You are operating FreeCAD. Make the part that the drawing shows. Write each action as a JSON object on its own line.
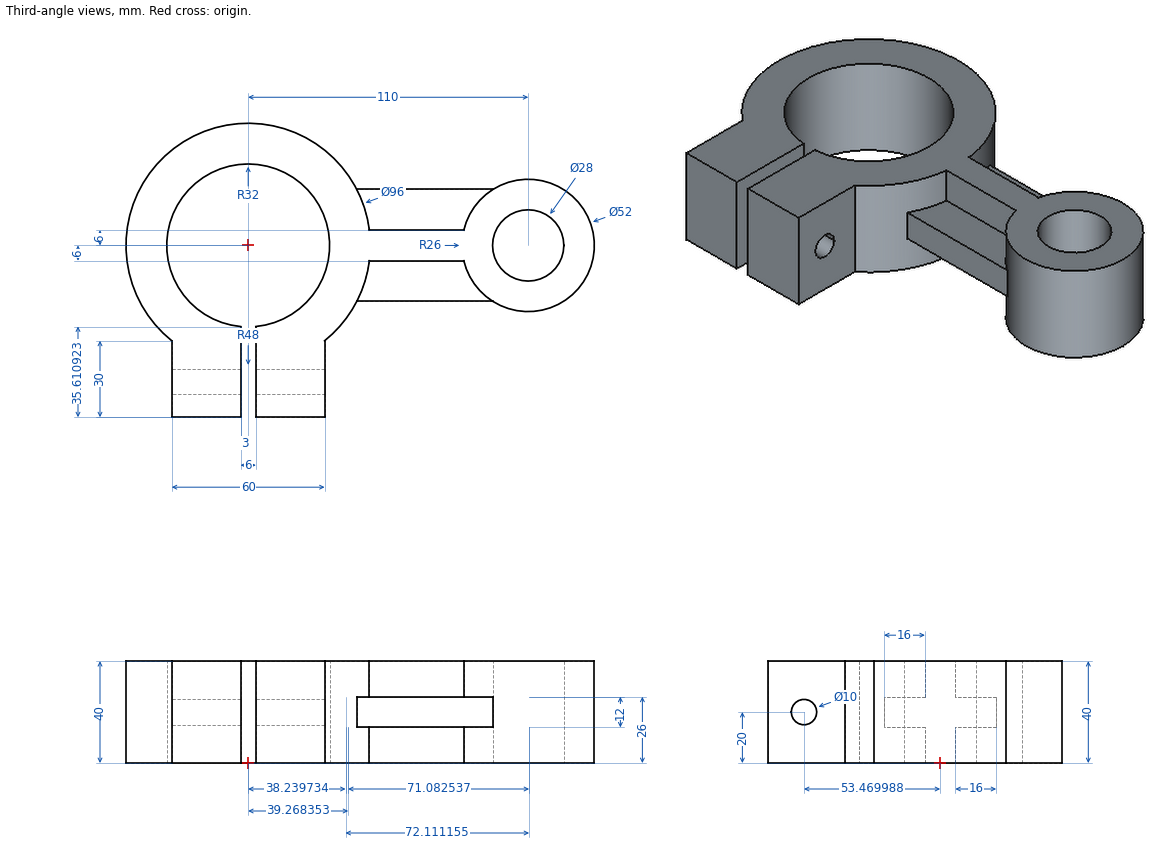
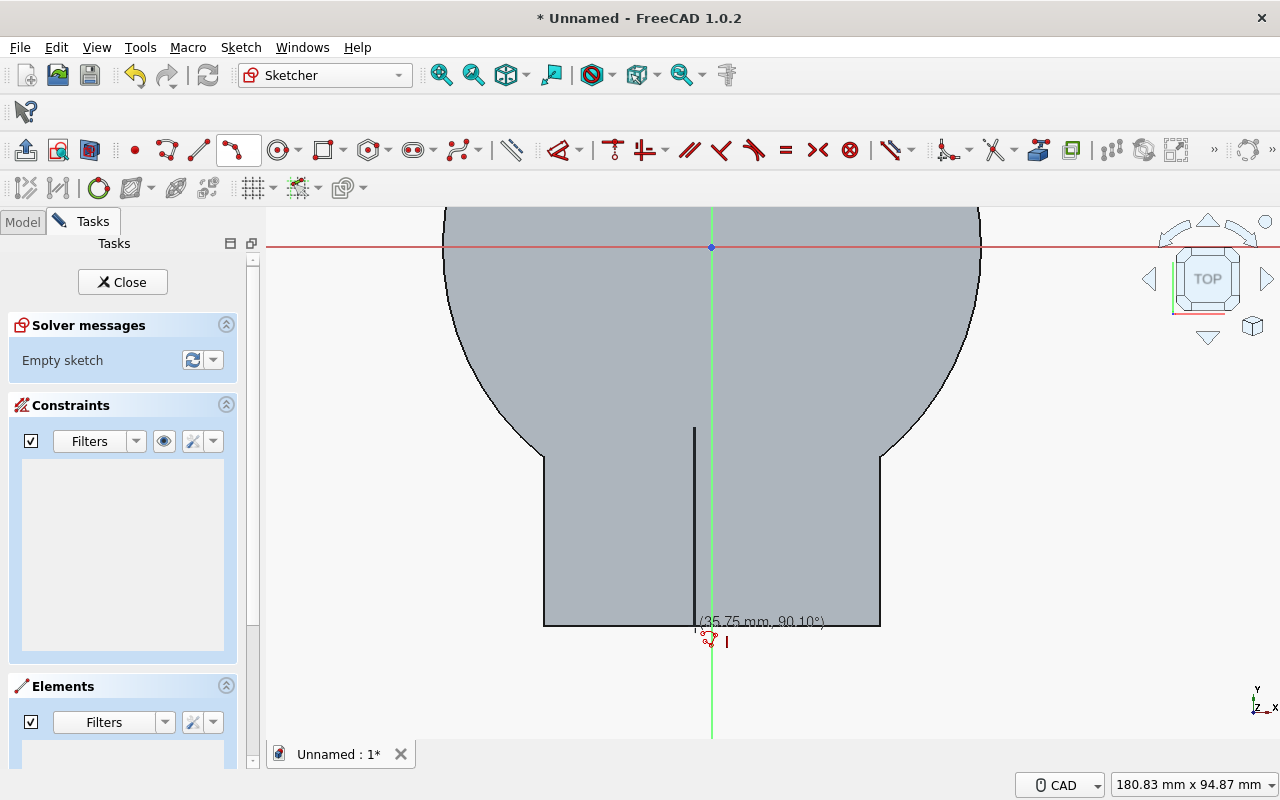
{"action": "left_click", "coordinate": [695, 626]}
{"action": "left_click", "coordinate": [729, 626]}
{"action": "left_click", "coordinate": [729, 426]}
{"action": "right_click", "coordinate": [729, 426]}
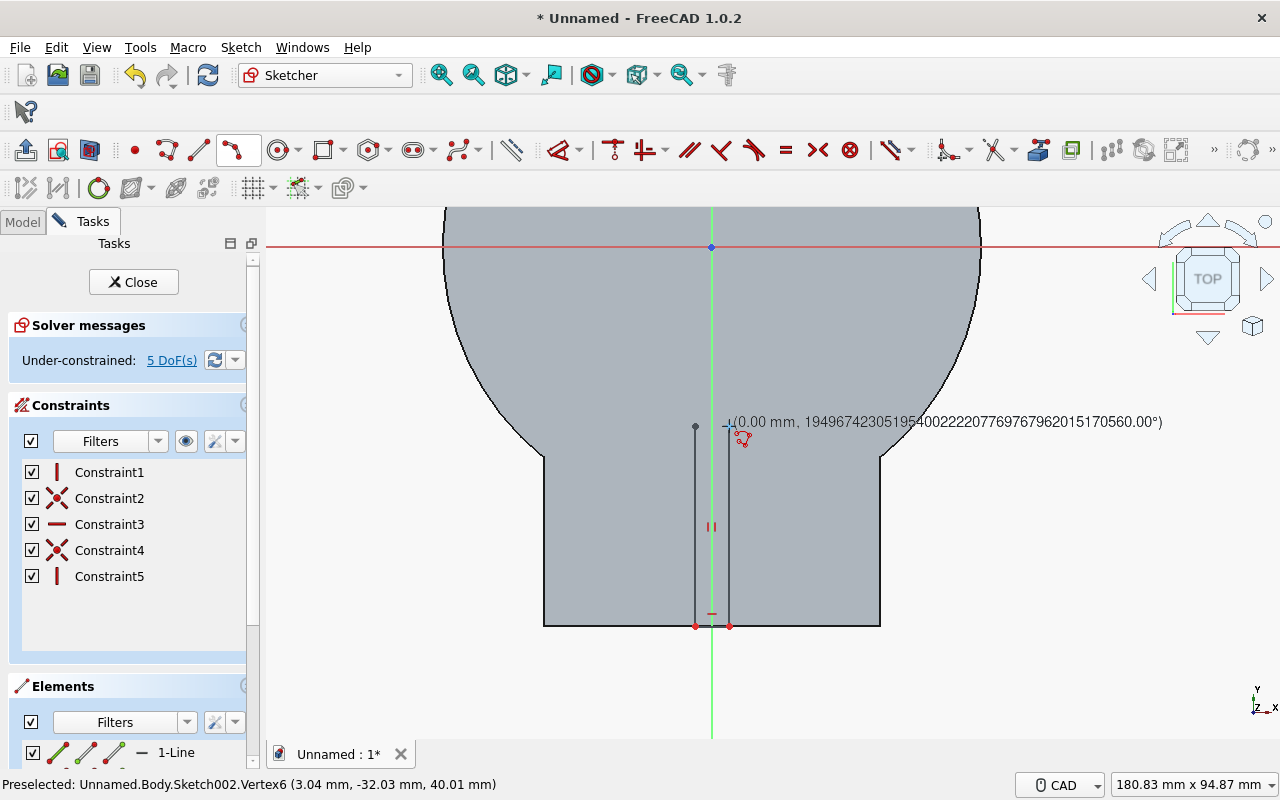
{"action": "left_click", "coordinate": [232, 150]}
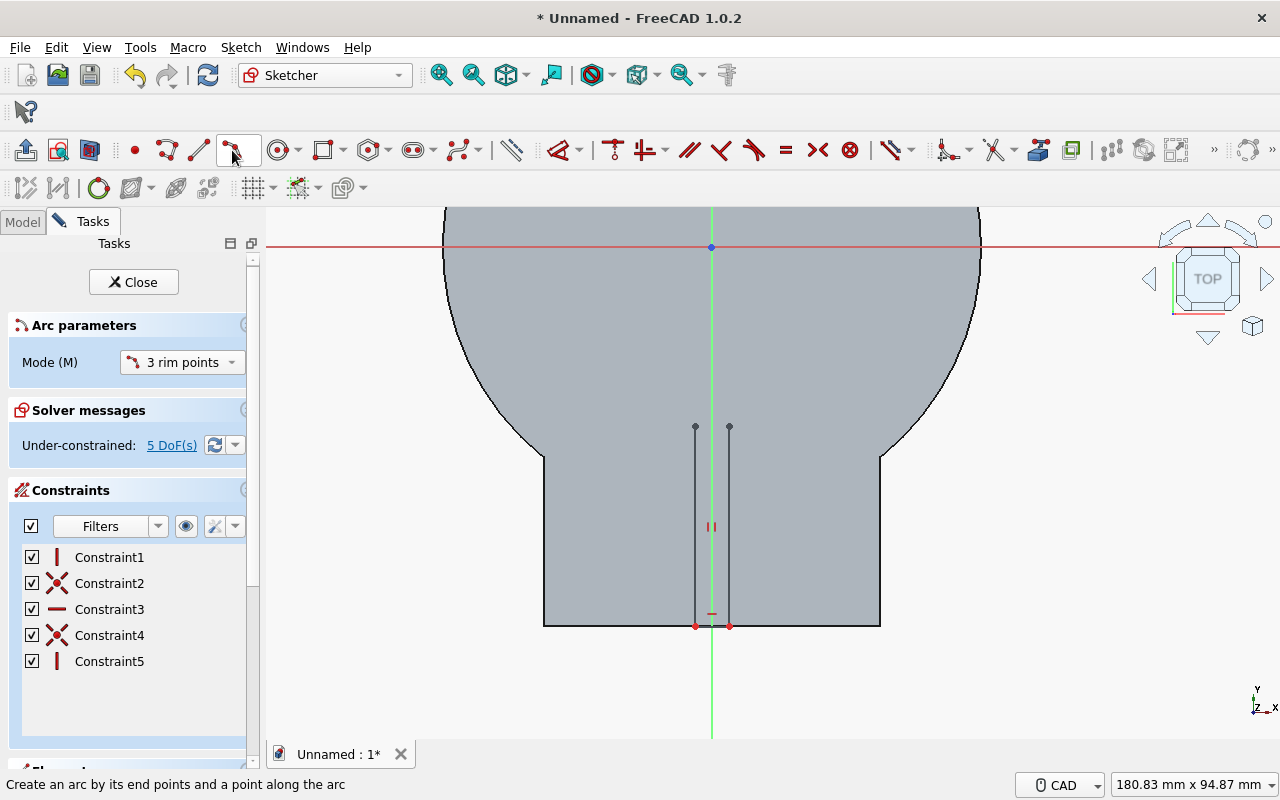
{"action": "left_click", "coordinate": [729, 427]}
{"action": "left_click", "coordinate": [695, 427]}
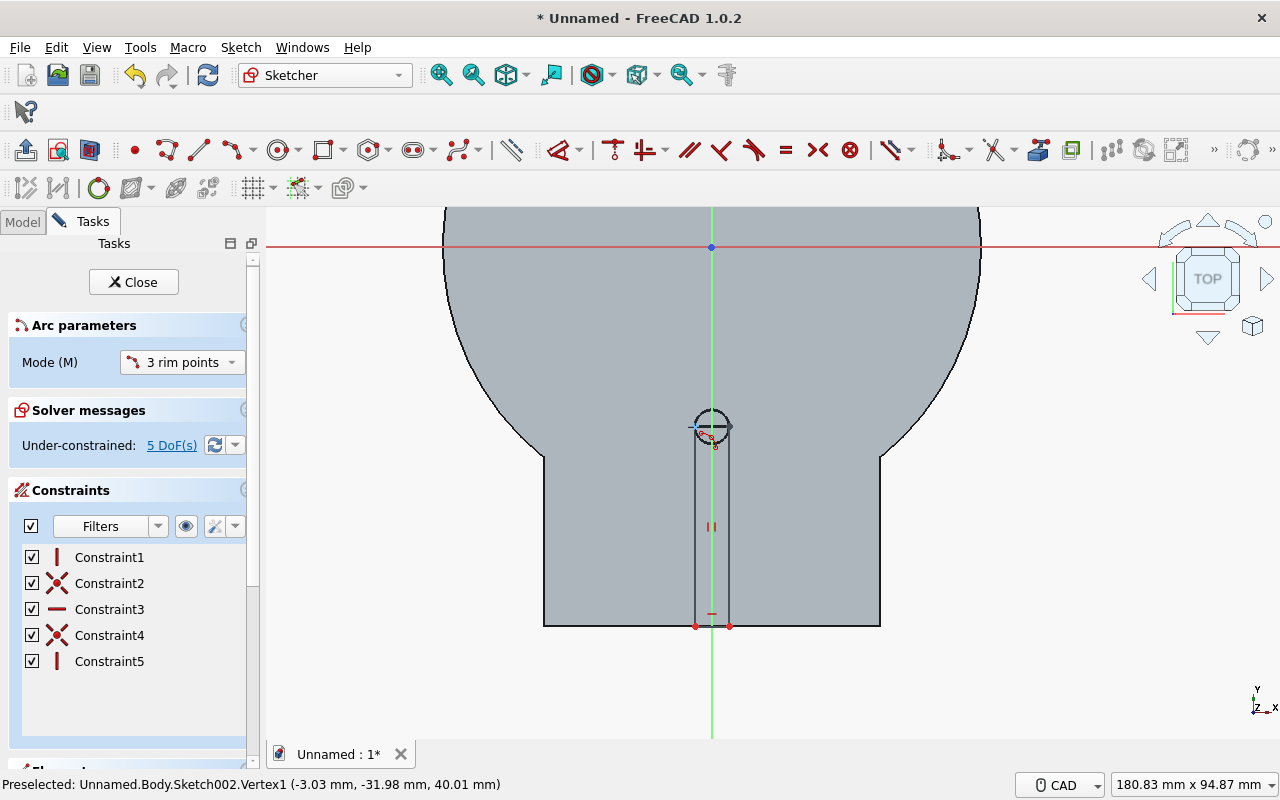
{"action": "scroll", "coordinate": [695, 626], "scroll_direction": "down", "scroll_amount": 3}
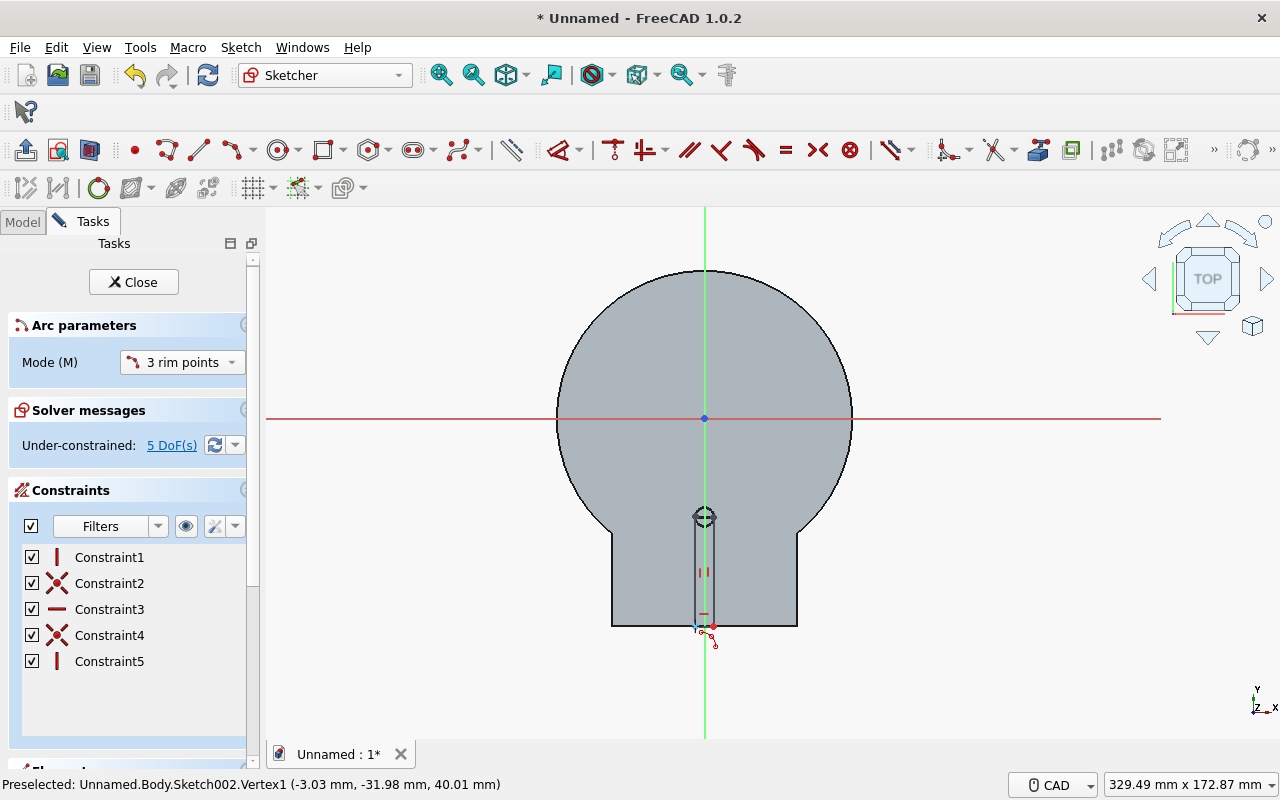
{"action": "left_click", "coordinate": [761, 338]}
{"action": "key", "text": "Escape"}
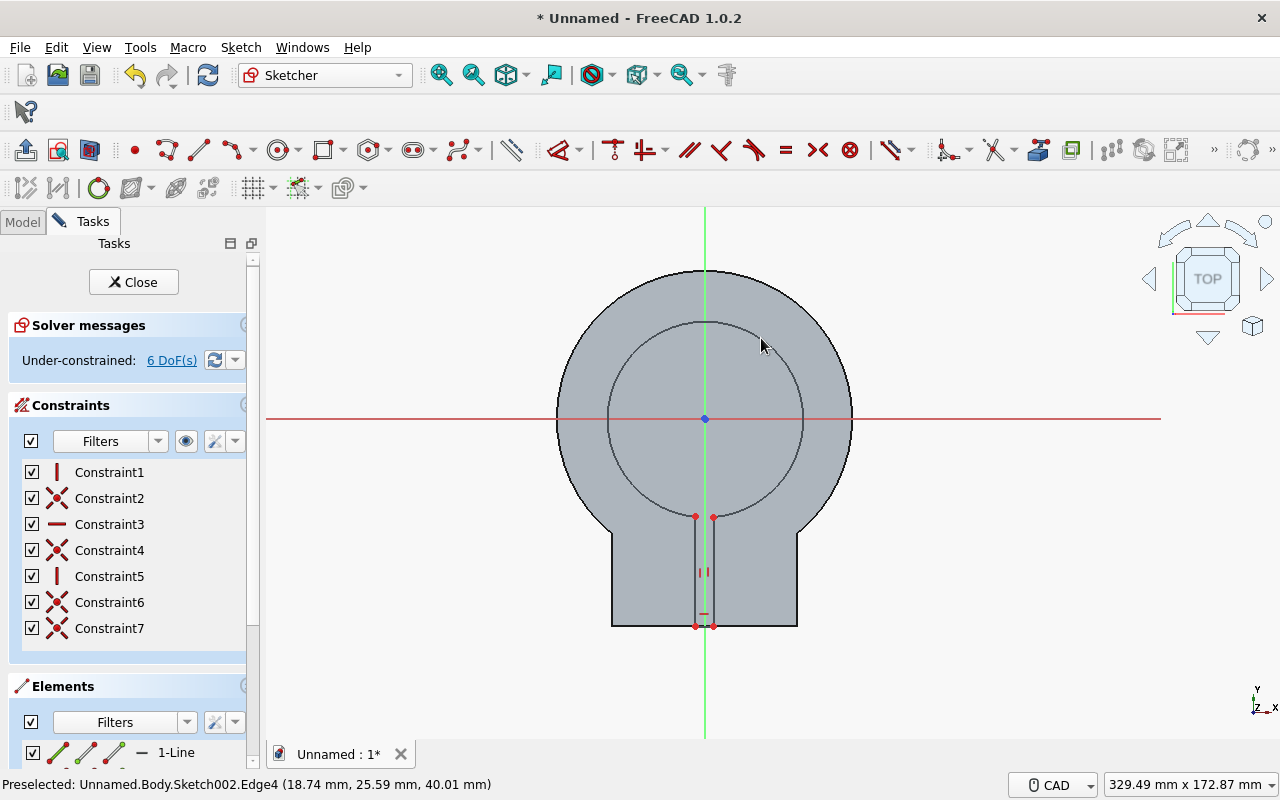
{"action": "left_click_drag", "start_coordinate": [695, 409], "coordinate": [715, 430]}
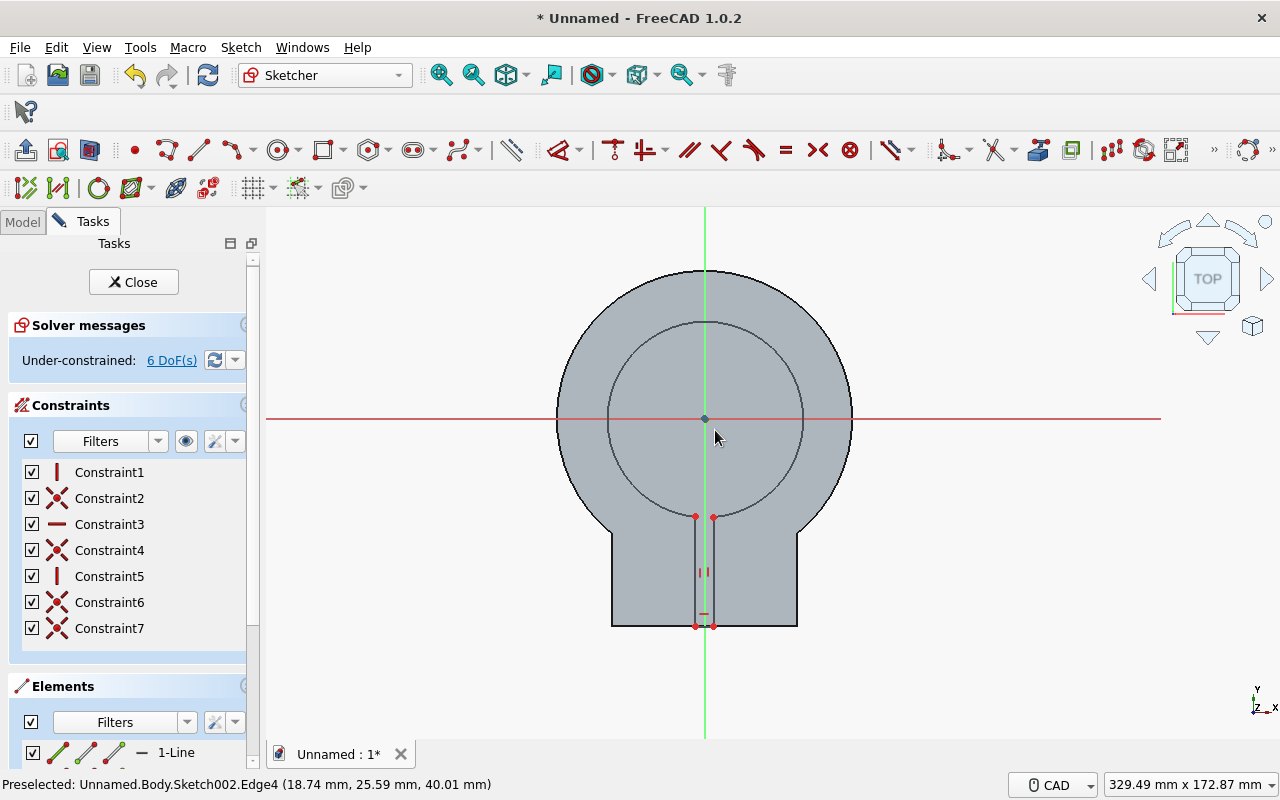
{"action": "left_click", "coordinate": [614, 150]}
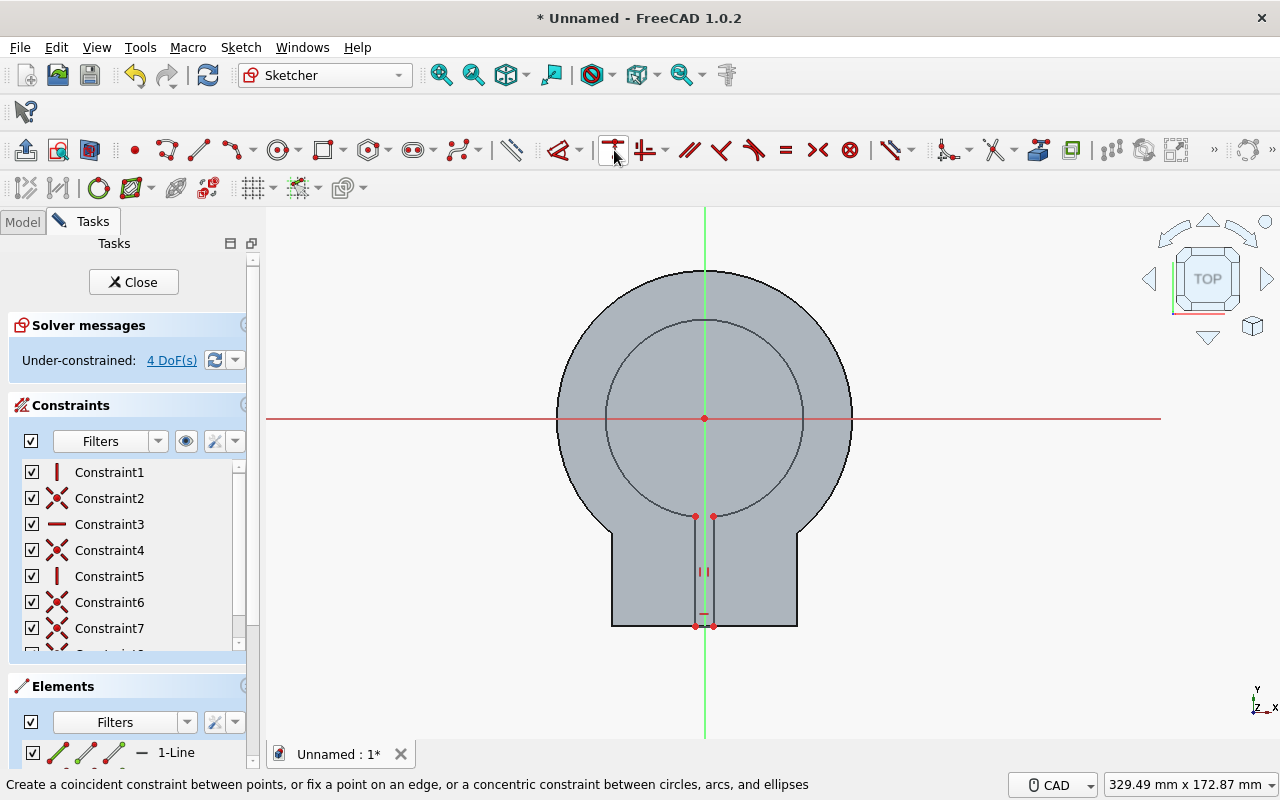
{"action": "left_click", "coordinate": [558, 150]}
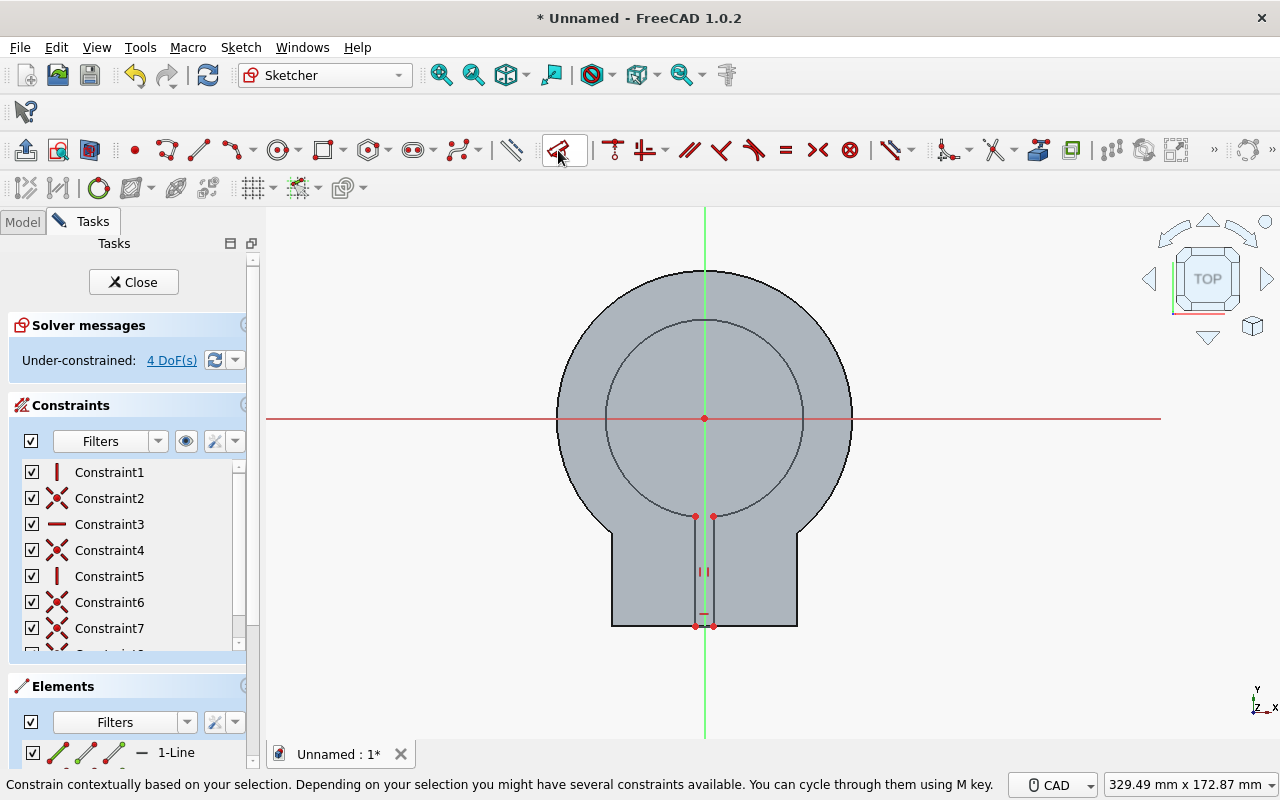
{"action": "left_click", "coordinate": [797, 384]}
{"action": "left_click", "coordinate": [827, 373]}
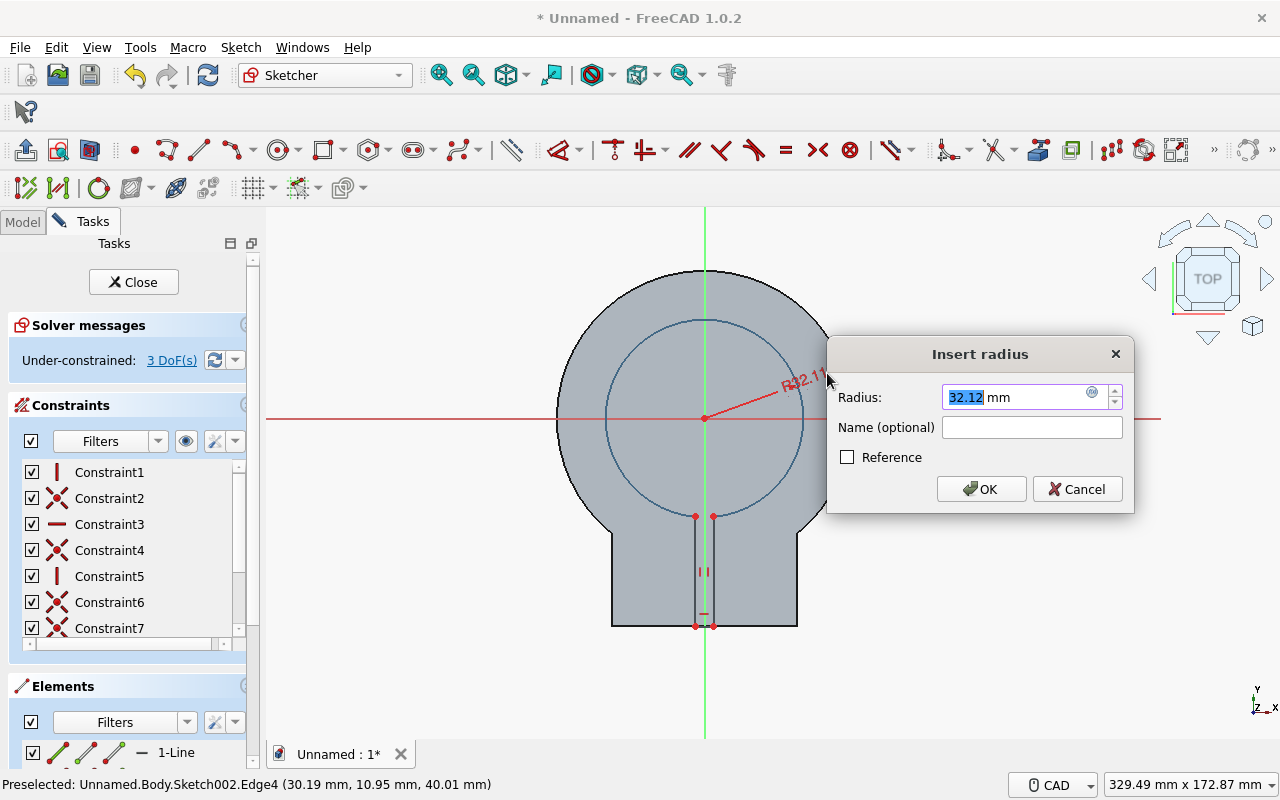
{"action": "type", "text": "32"}
{"action": "key", "text": "Return"}